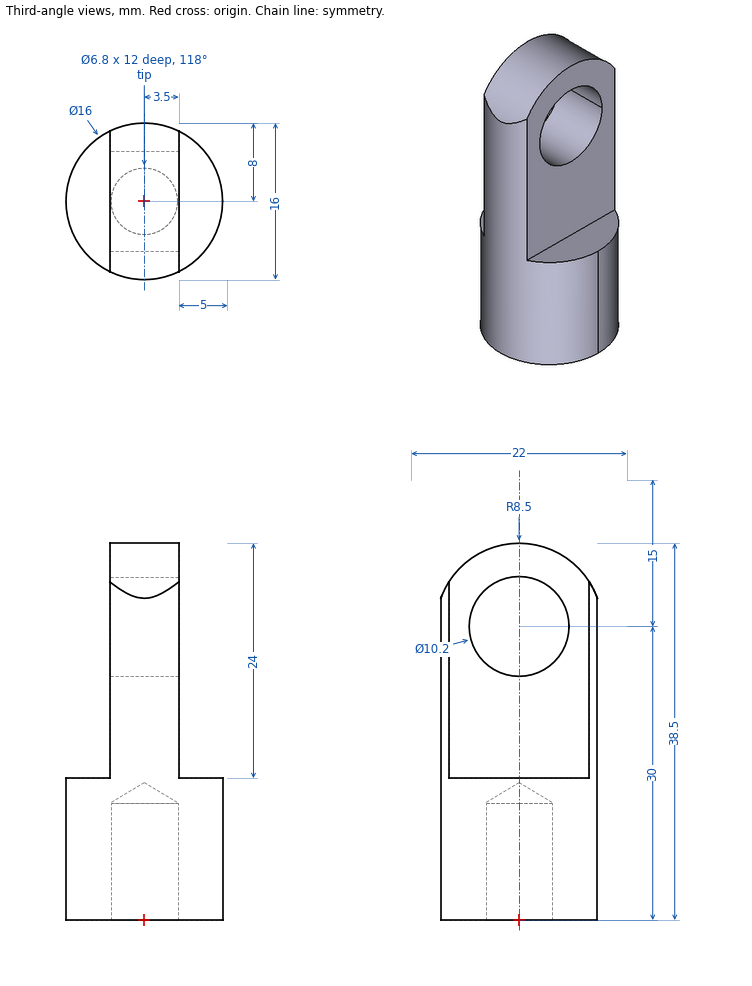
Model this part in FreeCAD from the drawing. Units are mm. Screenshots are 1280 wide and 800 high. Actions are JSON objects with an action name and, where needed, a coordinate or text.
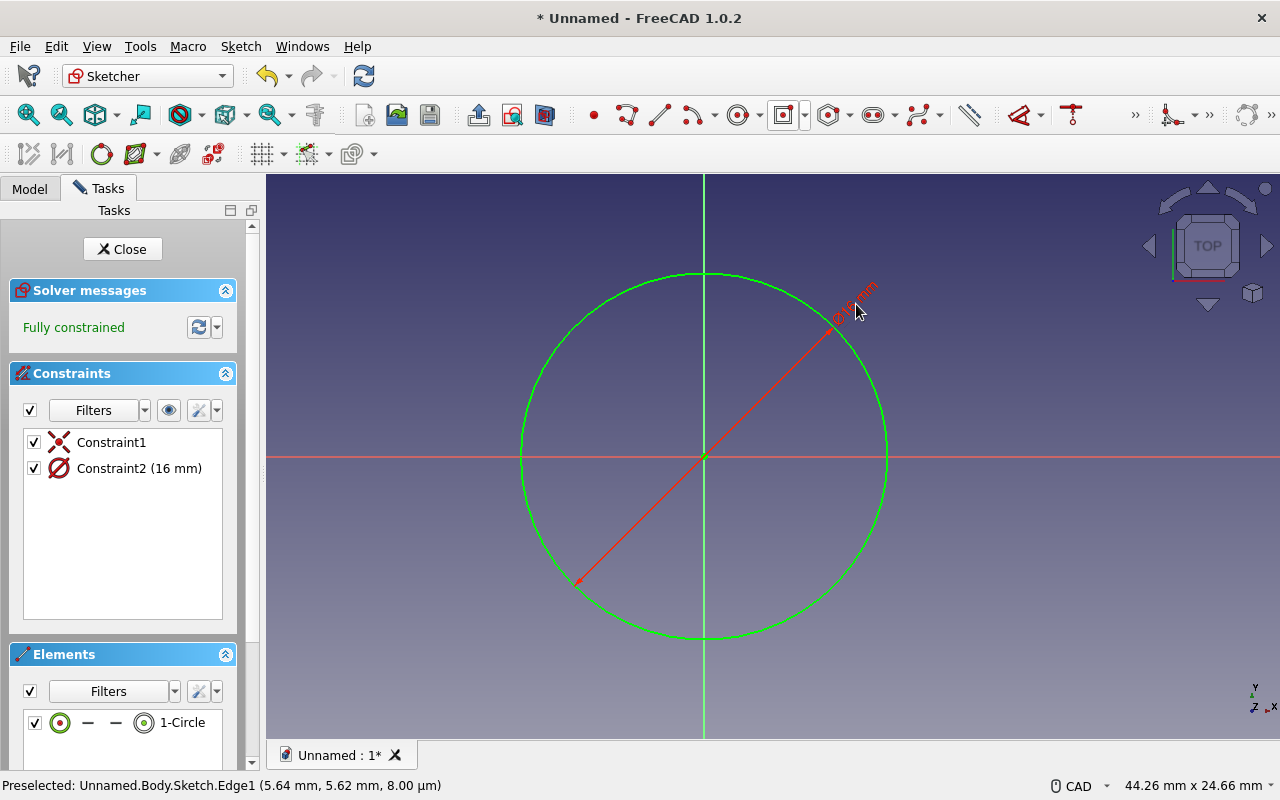
{"action": "left_click", "coordinate": [123, 249]}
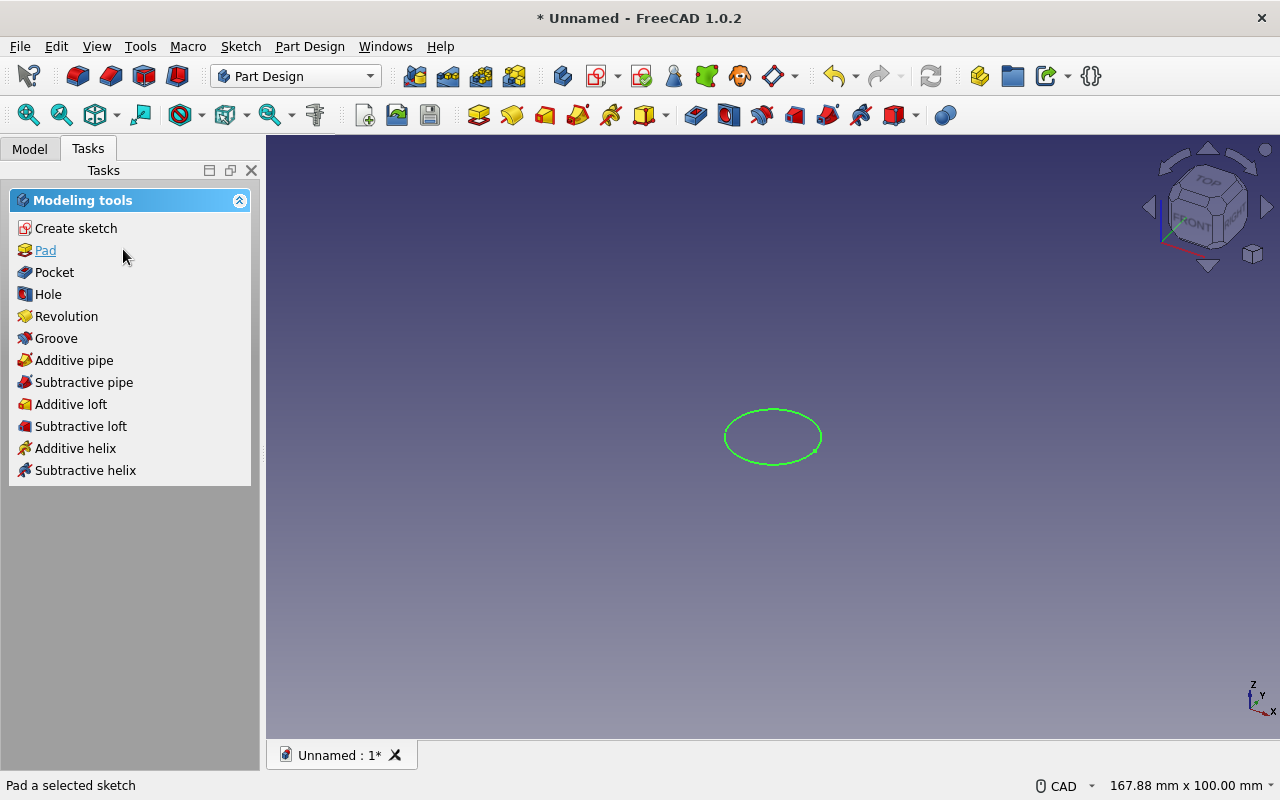
{"action": "left_click", "coordinate": [479, 116]}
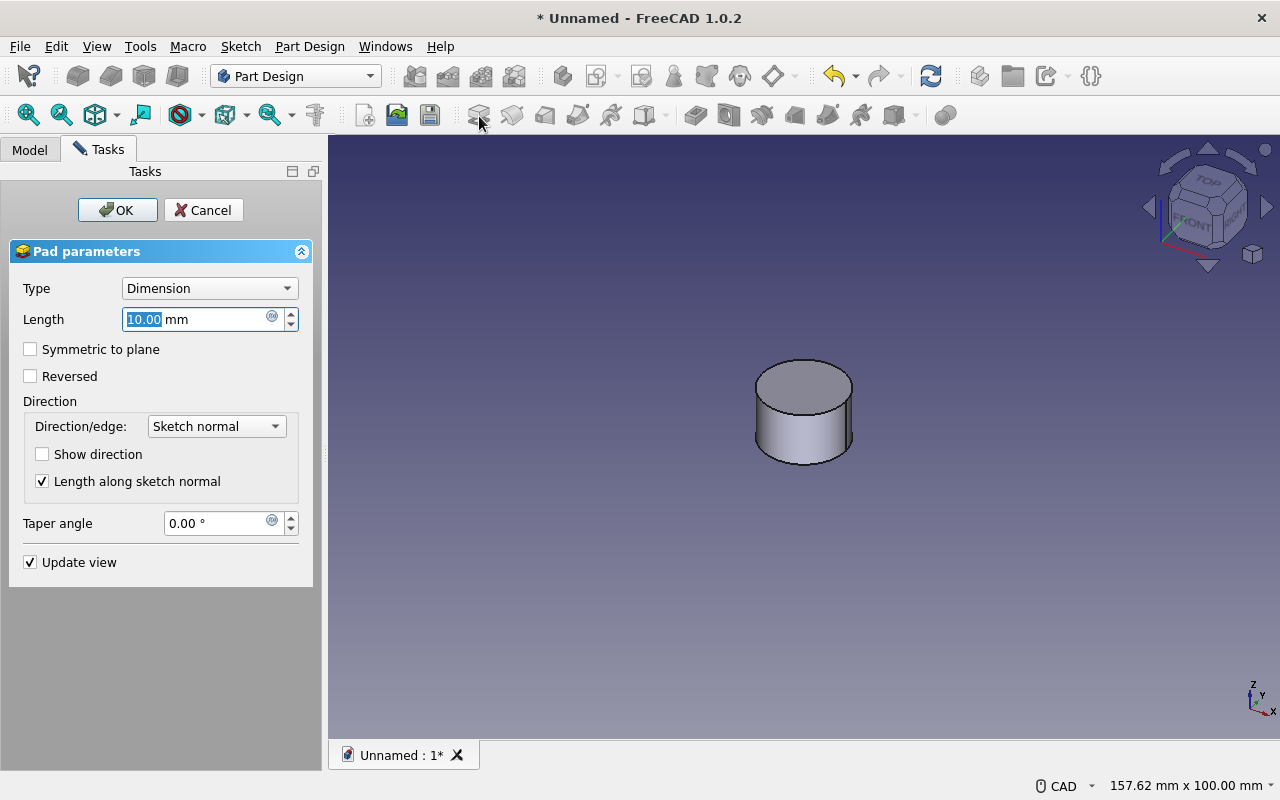
{"action": "type", "text": "38.5"}
{"action": "key", "text": "Tab"}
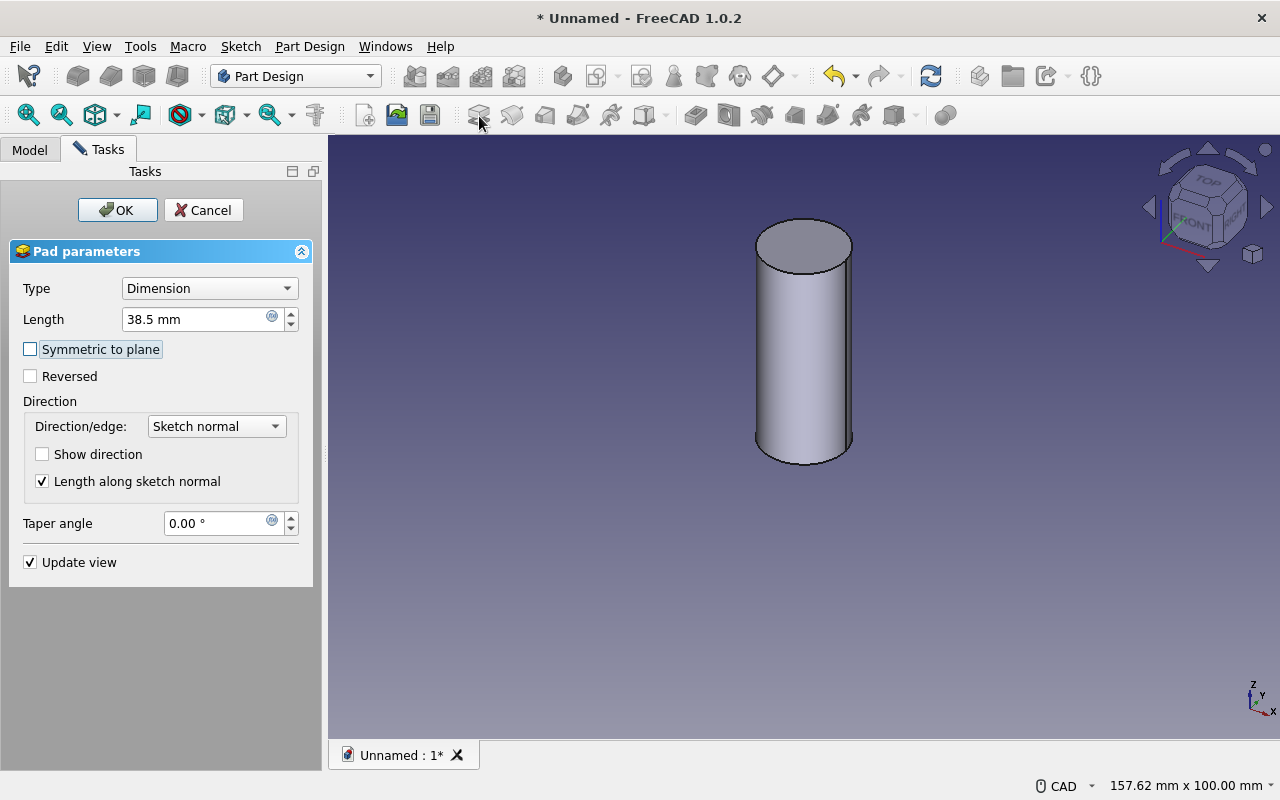
{"action": "left_click", "coordinate": [118, 210]}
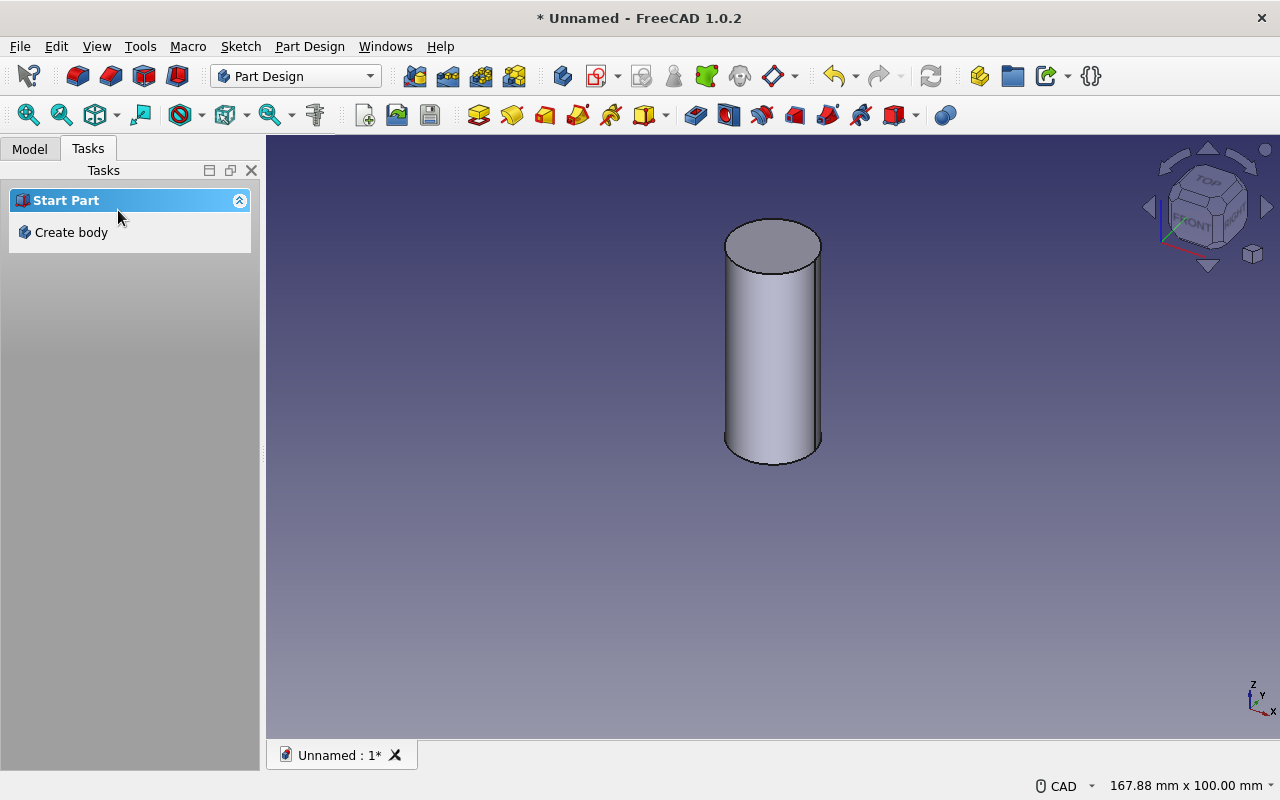
{"action": "key", "text": "v f"}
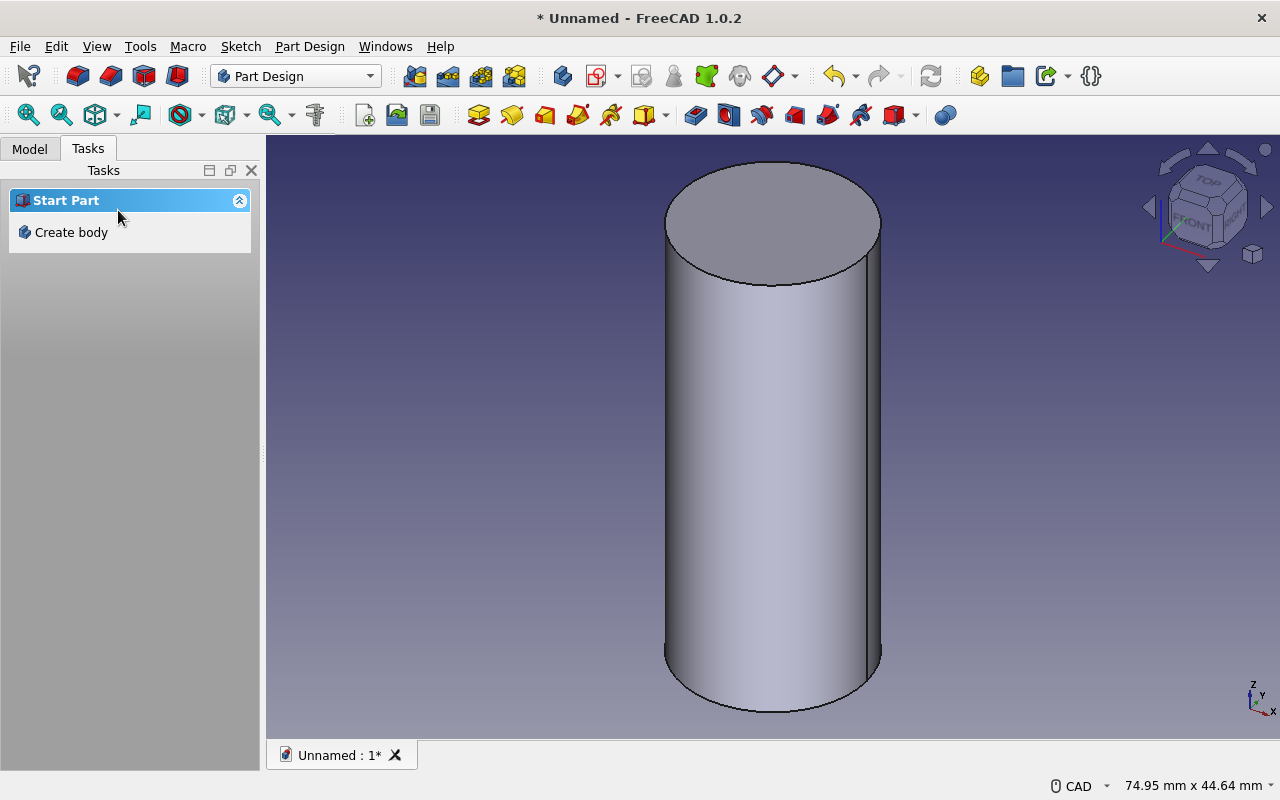
{"action": "left_click", "coordinate": [773, 223]}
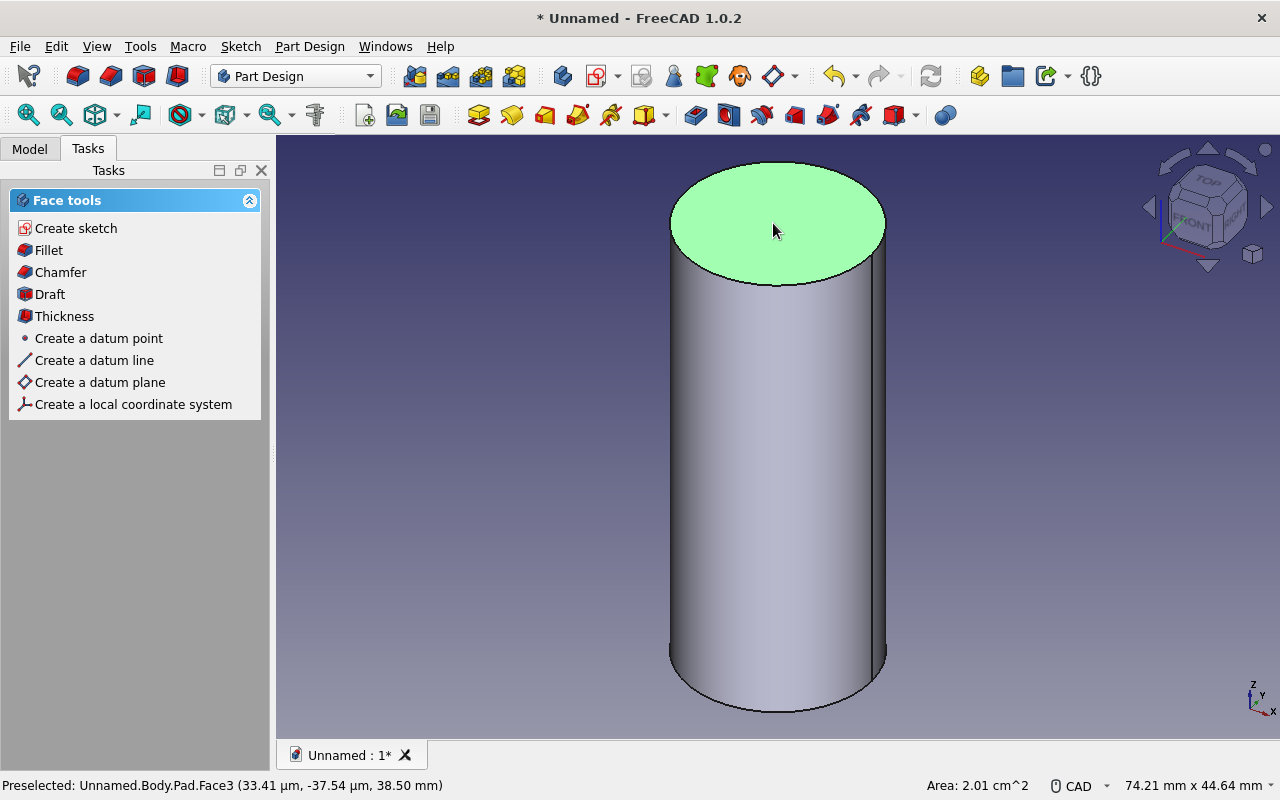
{"action": "left_click", "coordinate": [596, 76]}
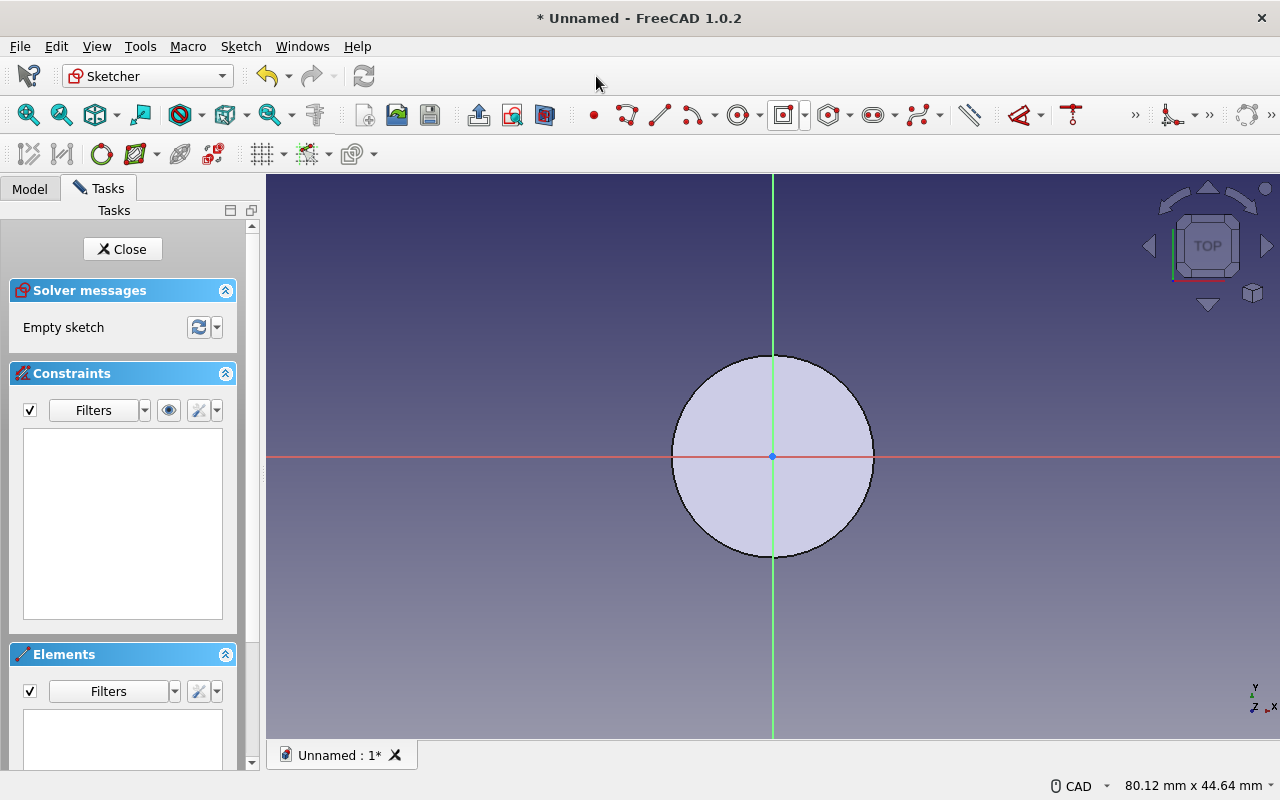
{"action": "scroll", "coordinate": [856, 456], "scroll_direction": "up", "scroll_amount": 3}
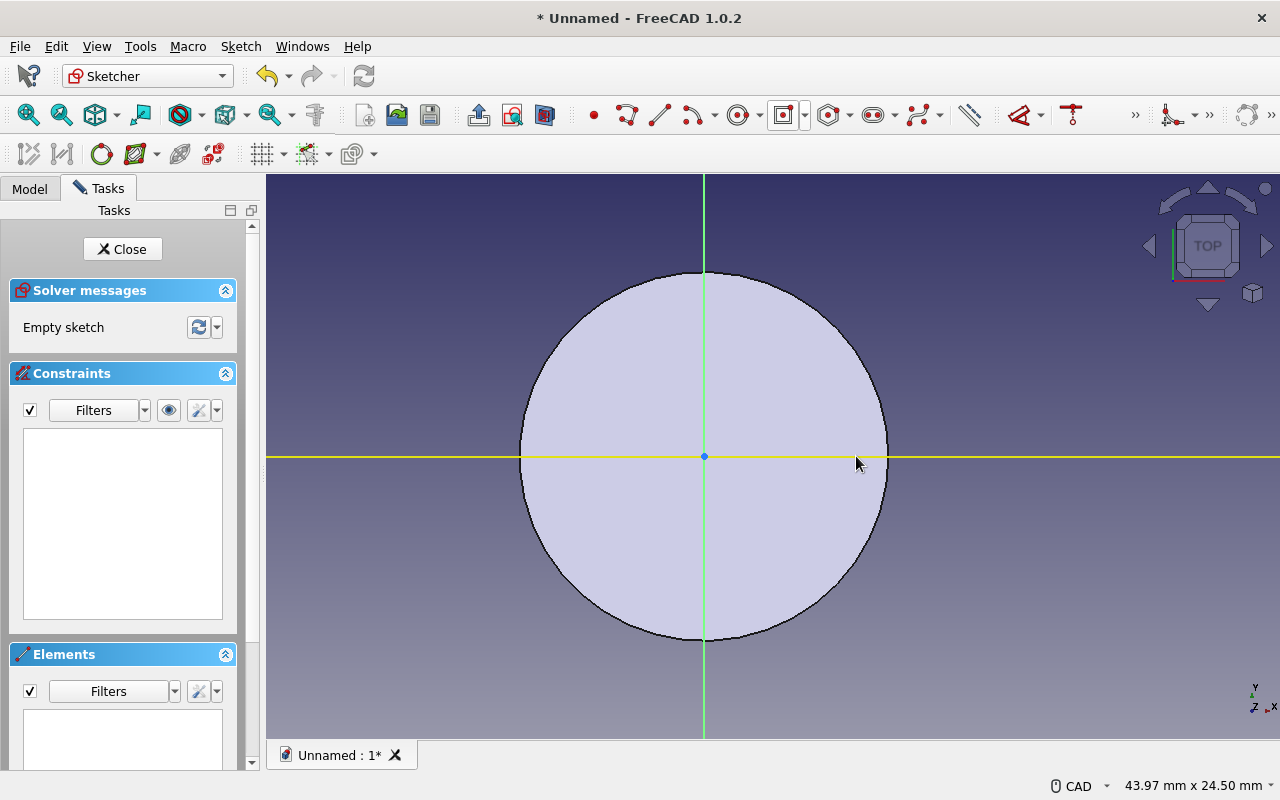
{"action": "left_click", "coordinate": [804, 116]}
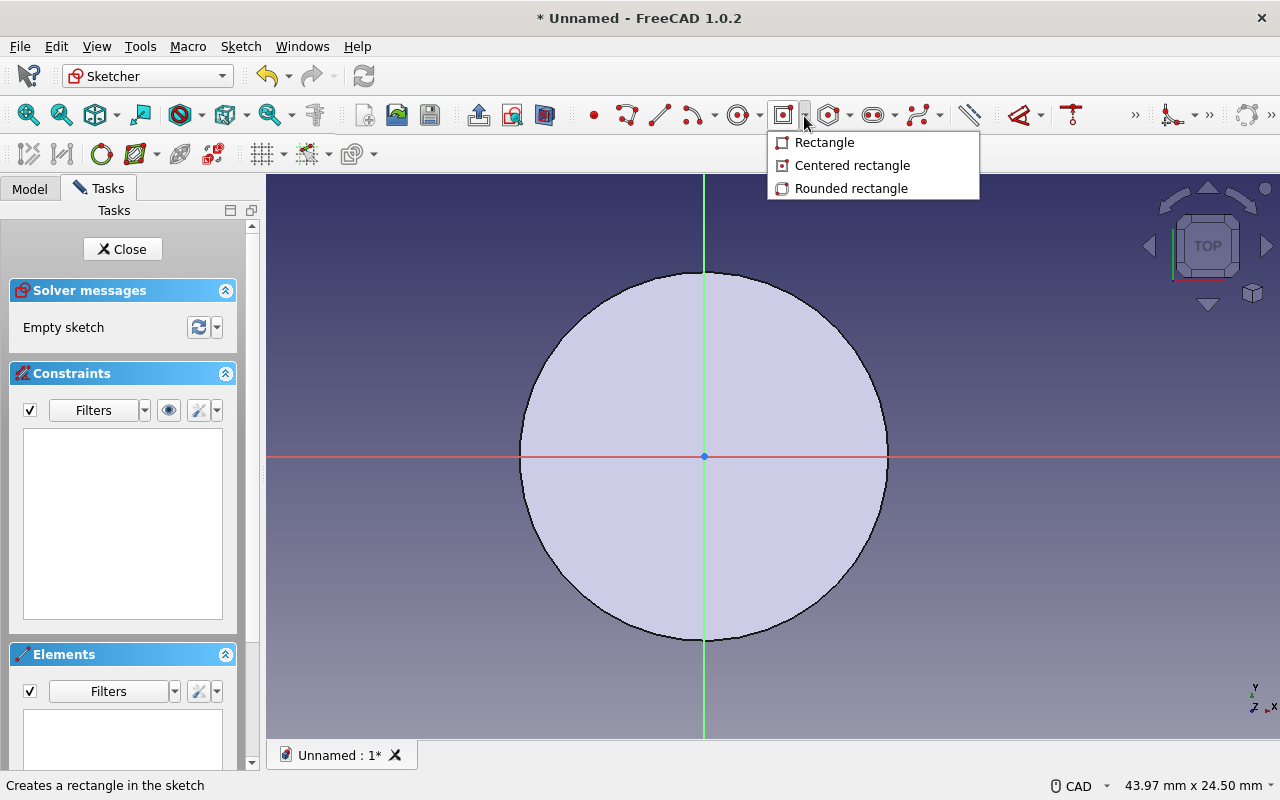
{"action": "left_click", "coordinate": [874, 142]}